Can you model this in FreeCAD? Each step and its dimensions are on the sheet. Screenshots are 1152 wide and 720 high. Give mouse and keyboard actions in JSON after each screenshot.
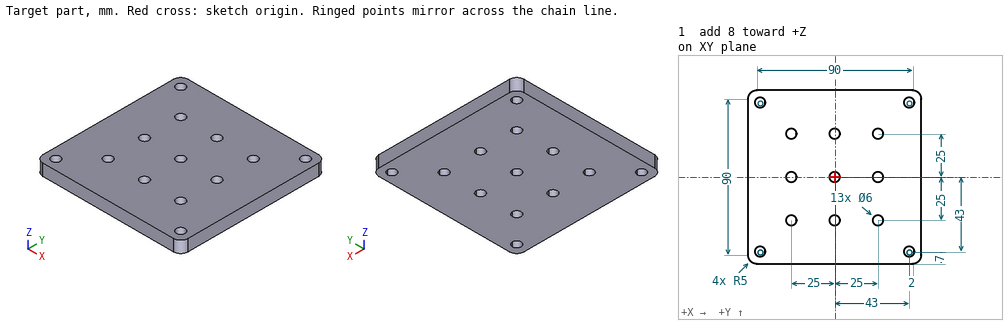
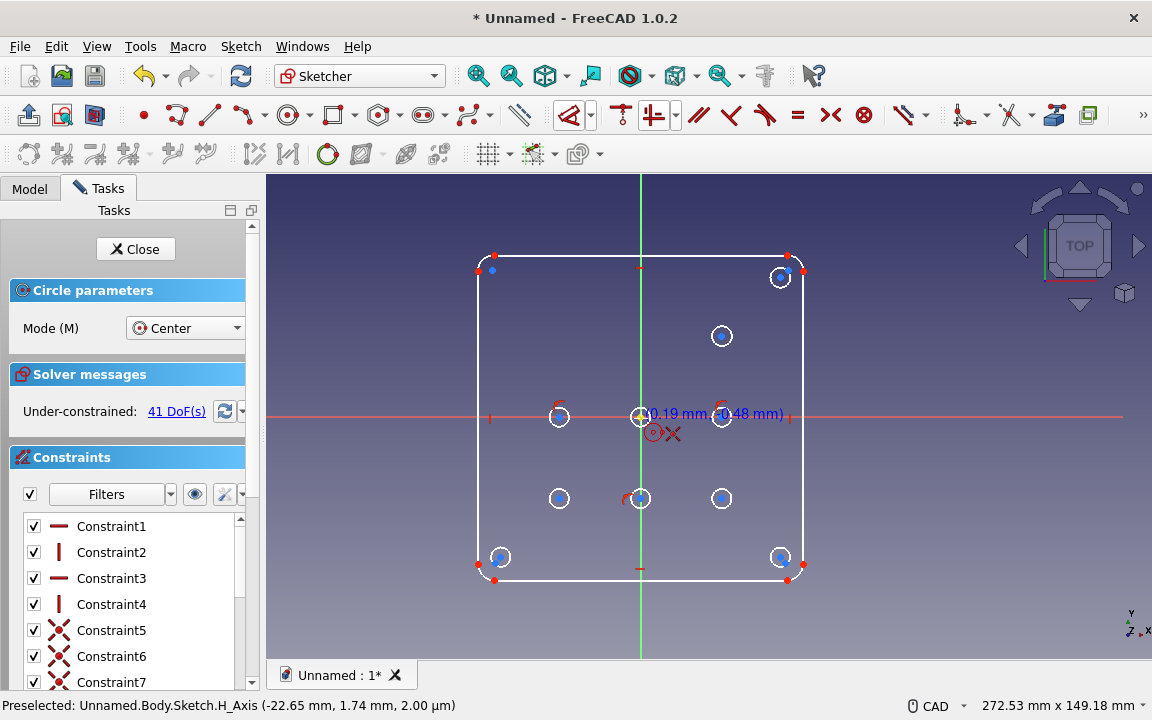
{"action": "scroll", "coordinate": [641, 336], "scroll_direction": "up", "scroll_amount": 5}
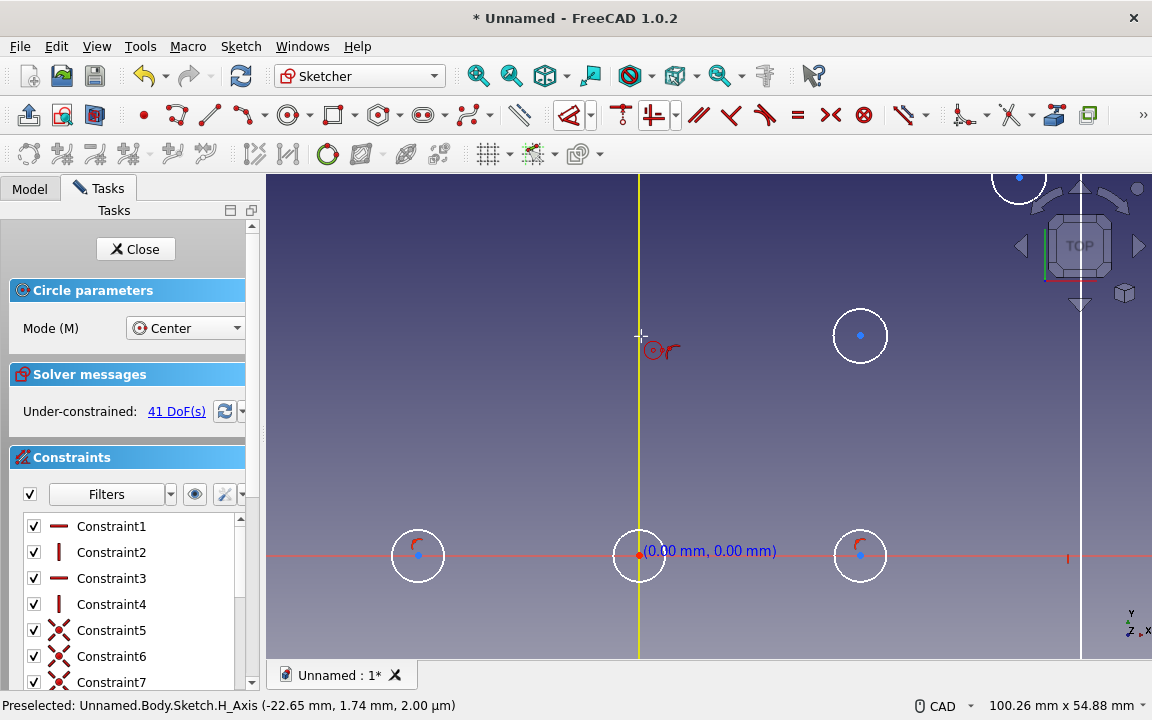
{"action": "left_click", "coordinate": [639, 335]}
{"action": "left_click", "coordinate": [658, 316]}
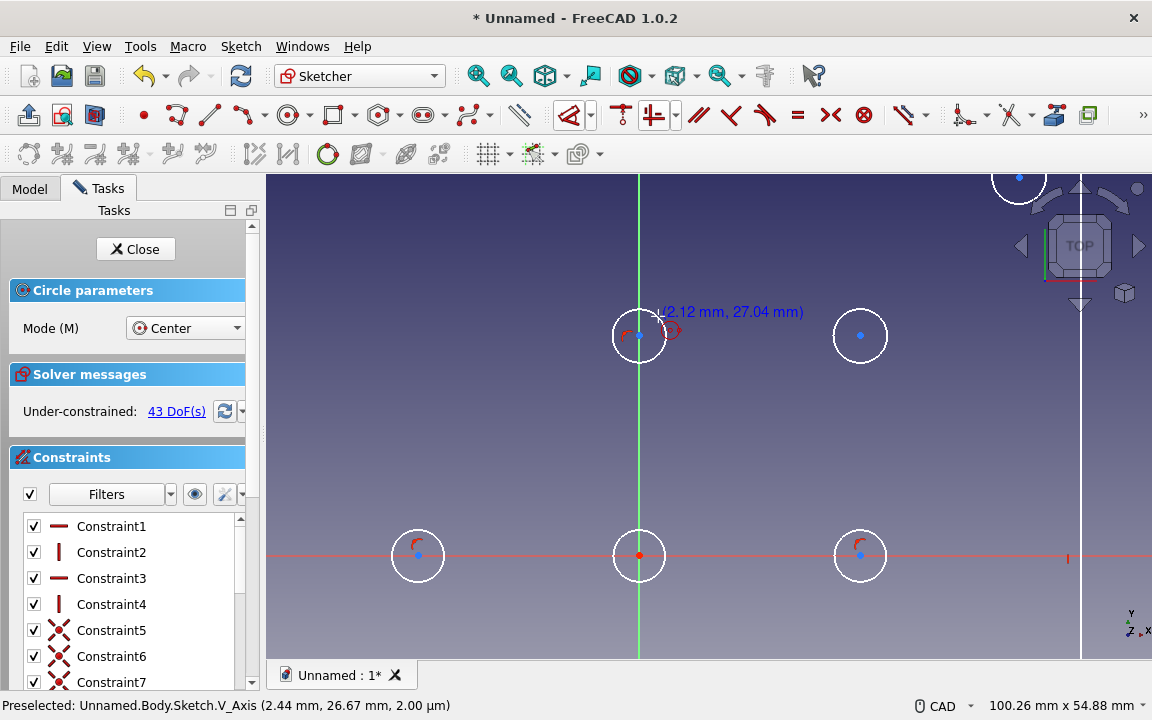
{"action": "left_click", "coordinate": [418, 335]}
{"action": "left_click", "coordinate": [437, 316]}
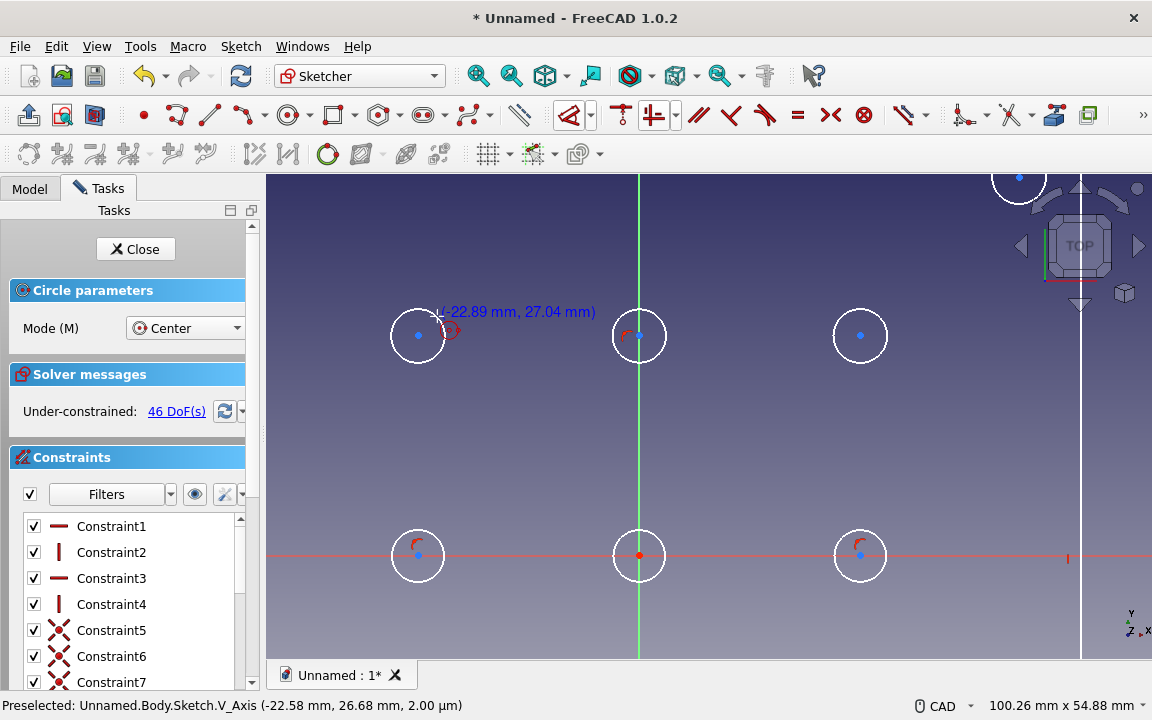
{"action": "scroll", "coordinate": [641, 335], "scroll_direction": "down", "scroll_amount": 5}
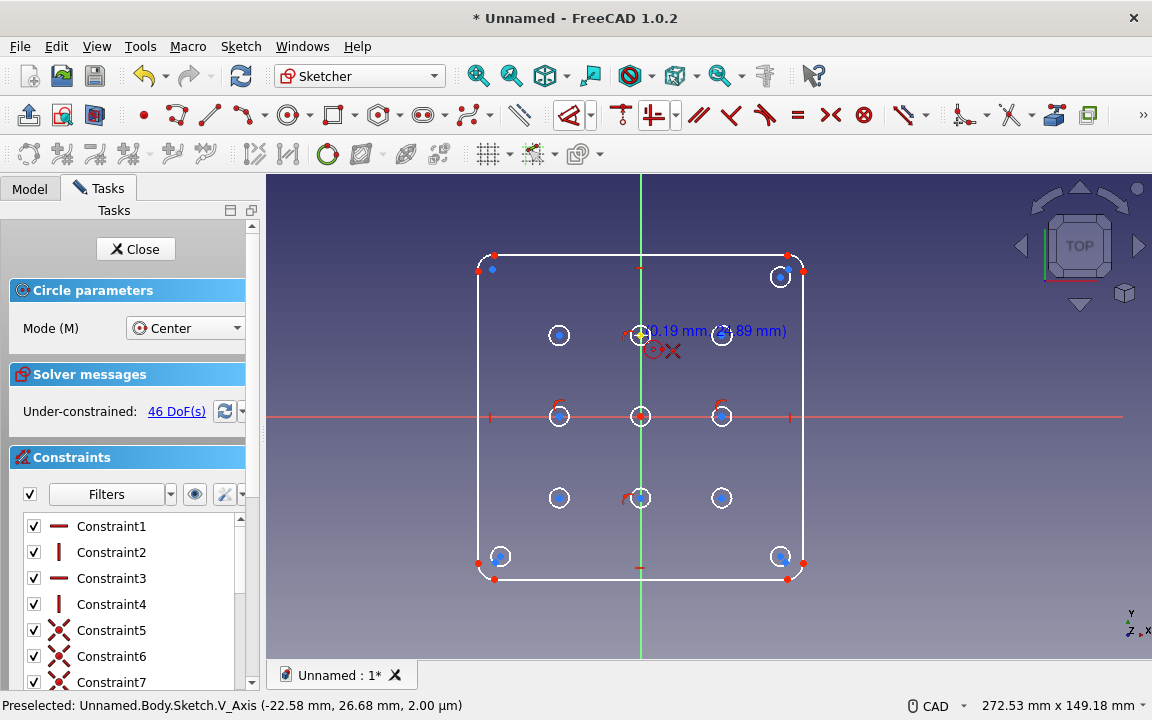
{"action": "scroll", "coordinate": [501, 277], "scroll_direction": "up", "scroll_amount": 5}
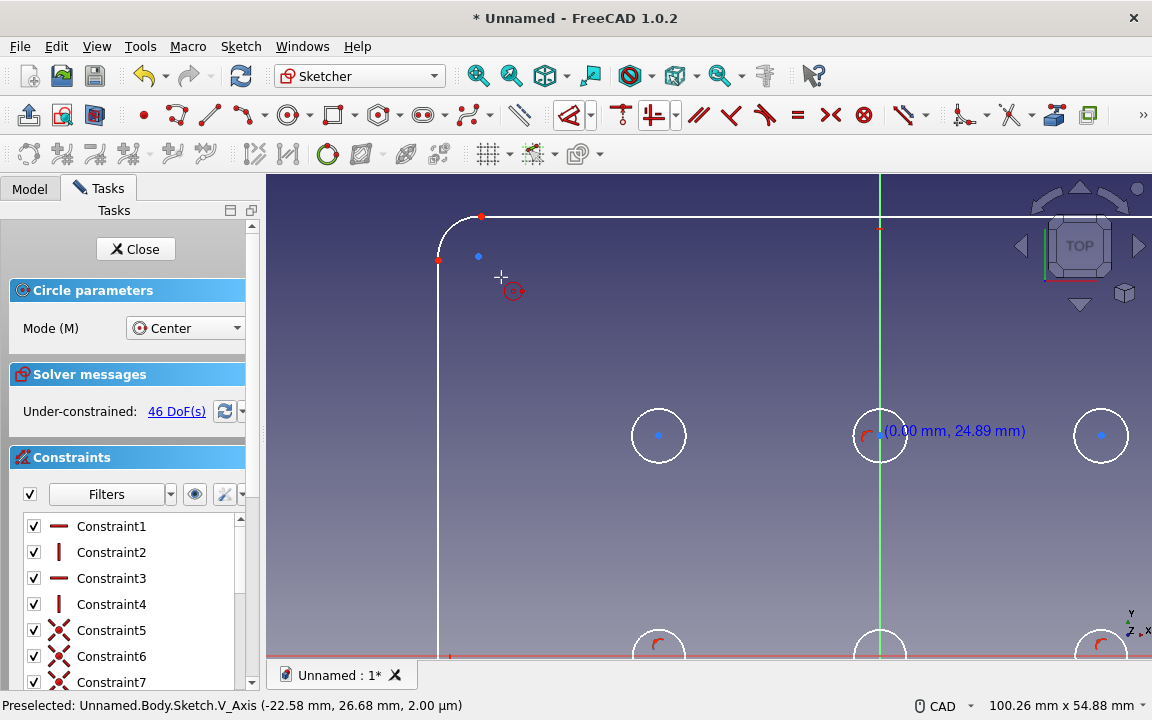
{"action": "left_click", "coordinate": [500, 276]}
{"action": "left_click", "coordinate": [519, 257]}
{"action": "key", "text": "Escape"}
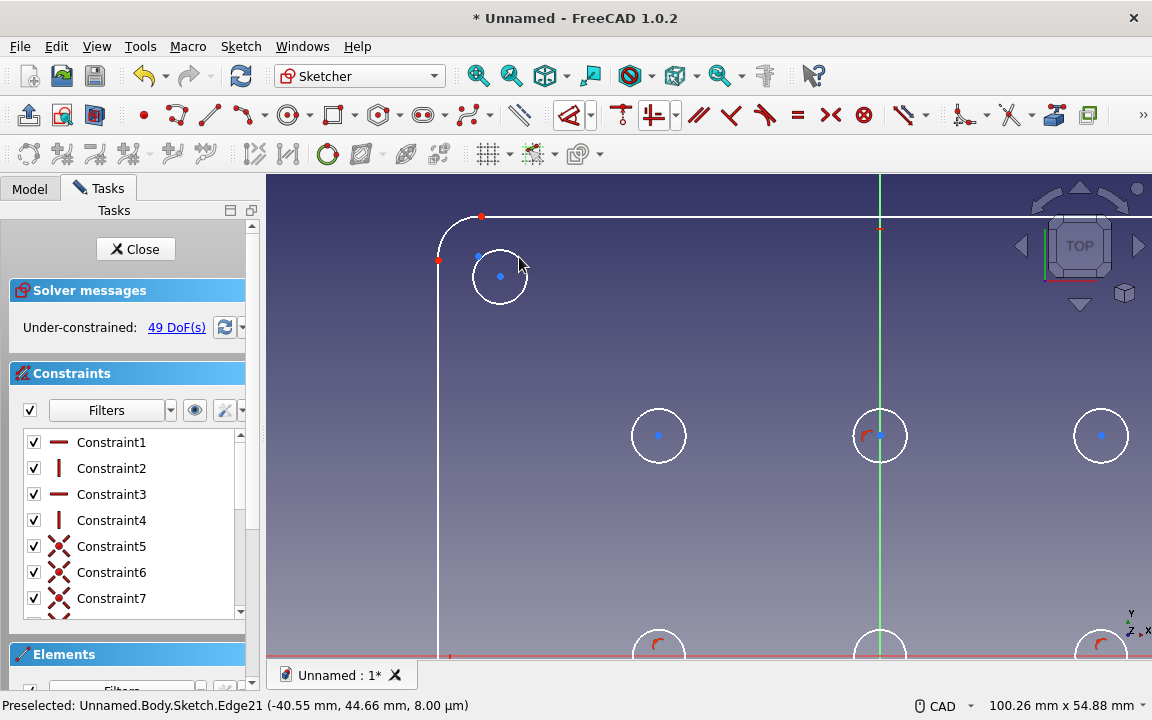
{"action": "left_click", "coordinate": [721, 217]}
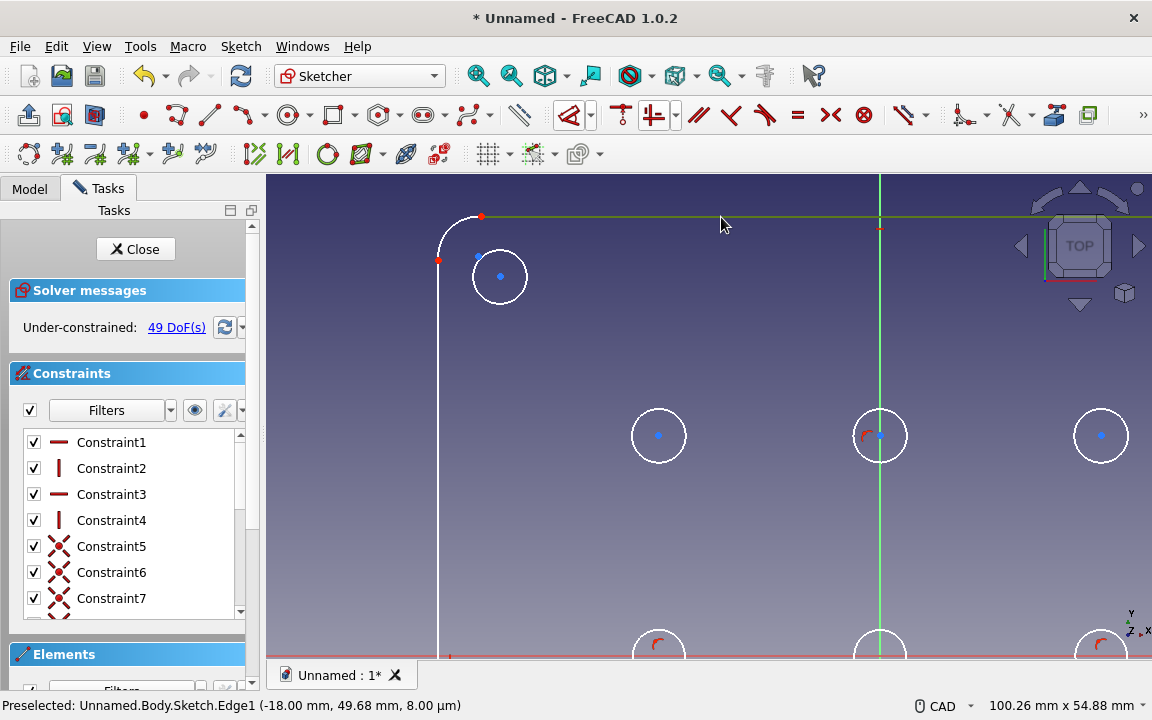
{"action": "left_click", "coordinate": [461, 220]}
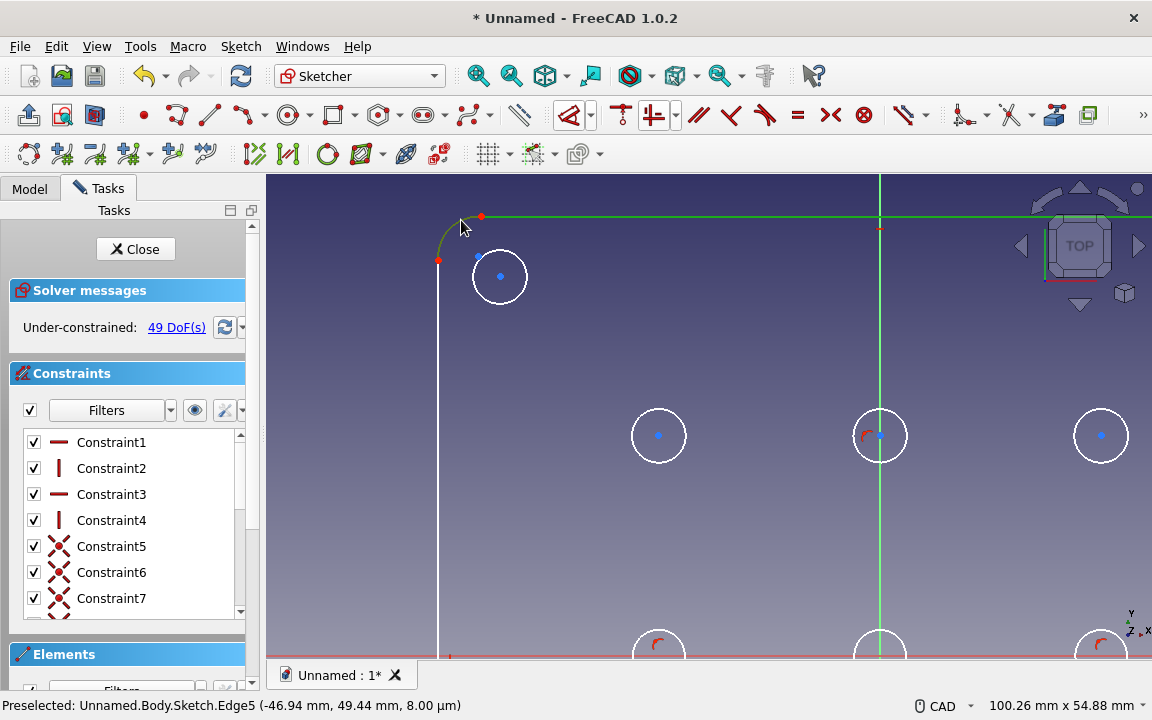
{"action": "left_click", "coordinate": [765, 116]}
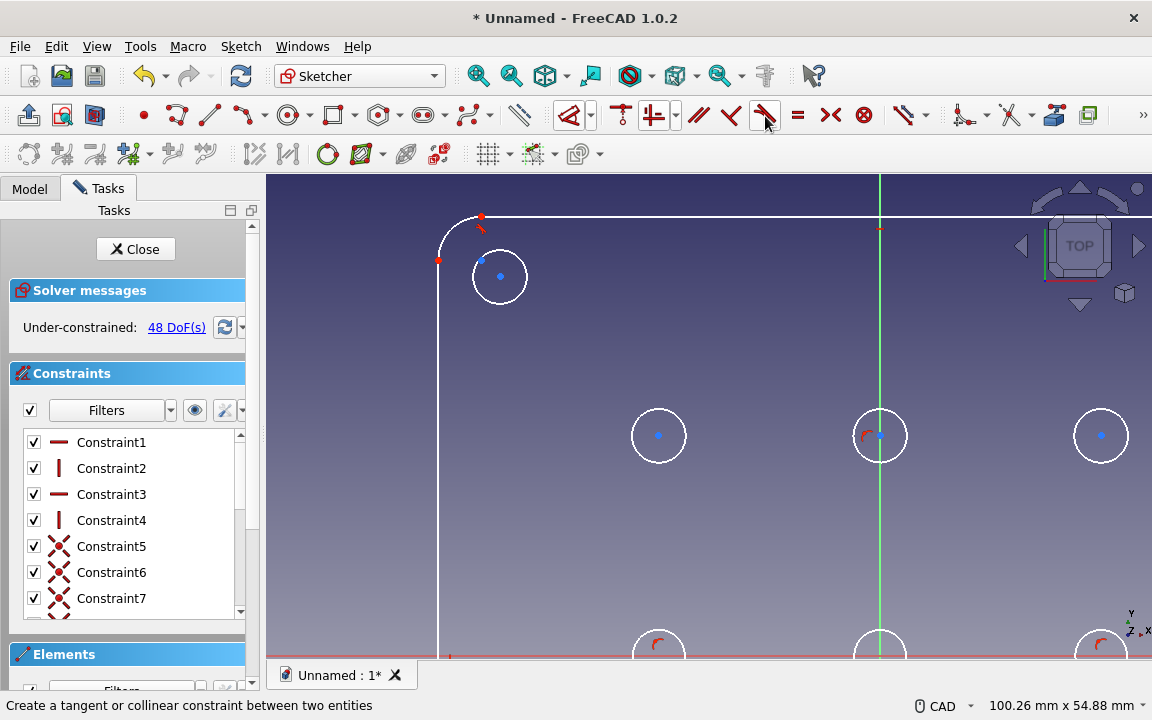
{"action": "left_click", "coordinate": [721, 217]}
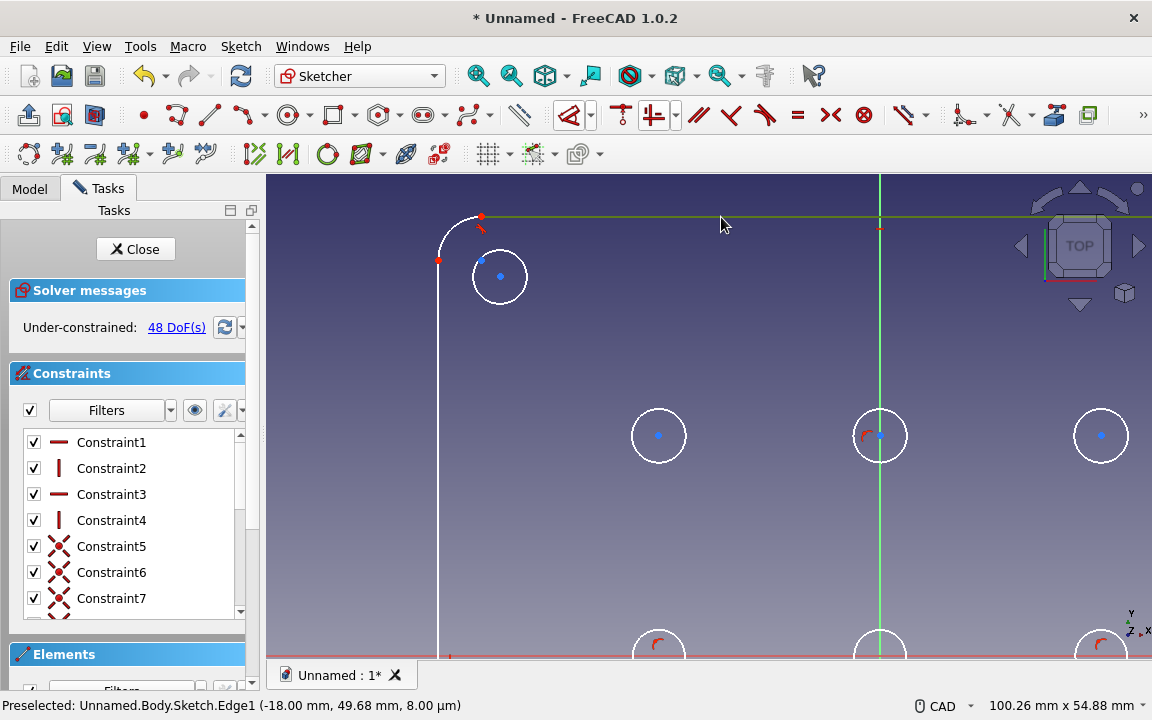
{"action": "scroll", "coordinate": [501, 277], "scroll_direction": "down", "scroll_amount": 5}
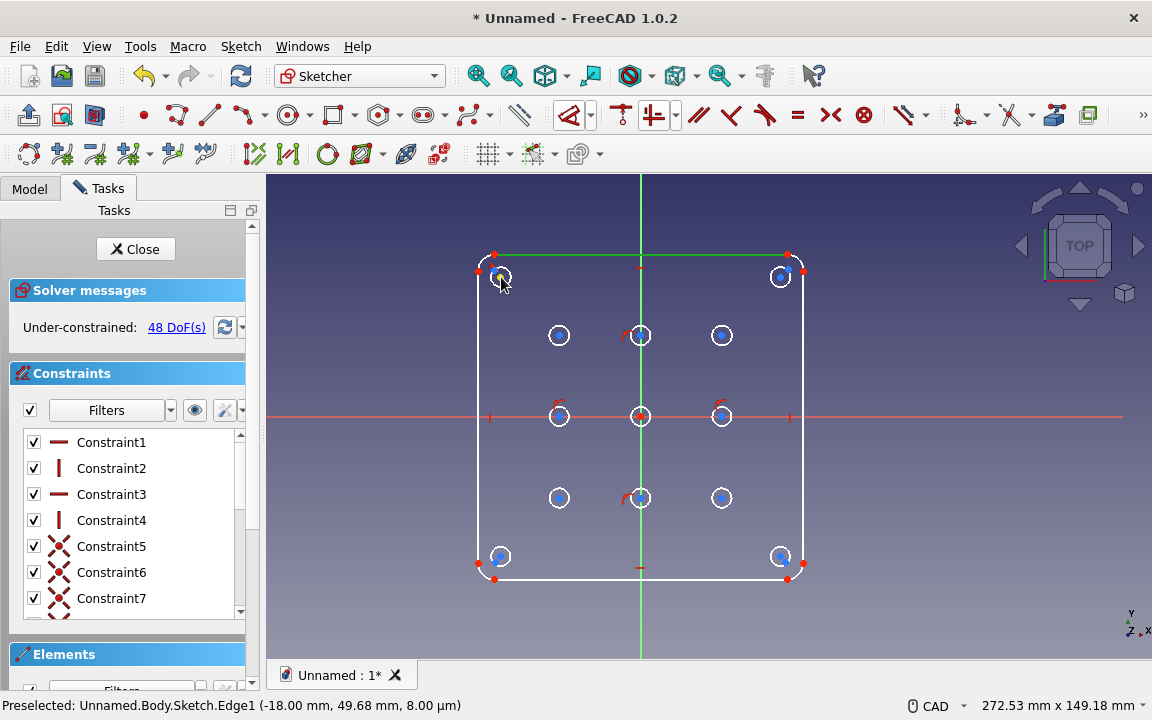
{"action": "scroll", "coordinate": [802, 264], "scroll_direction": "up", "scroll_amount": 3}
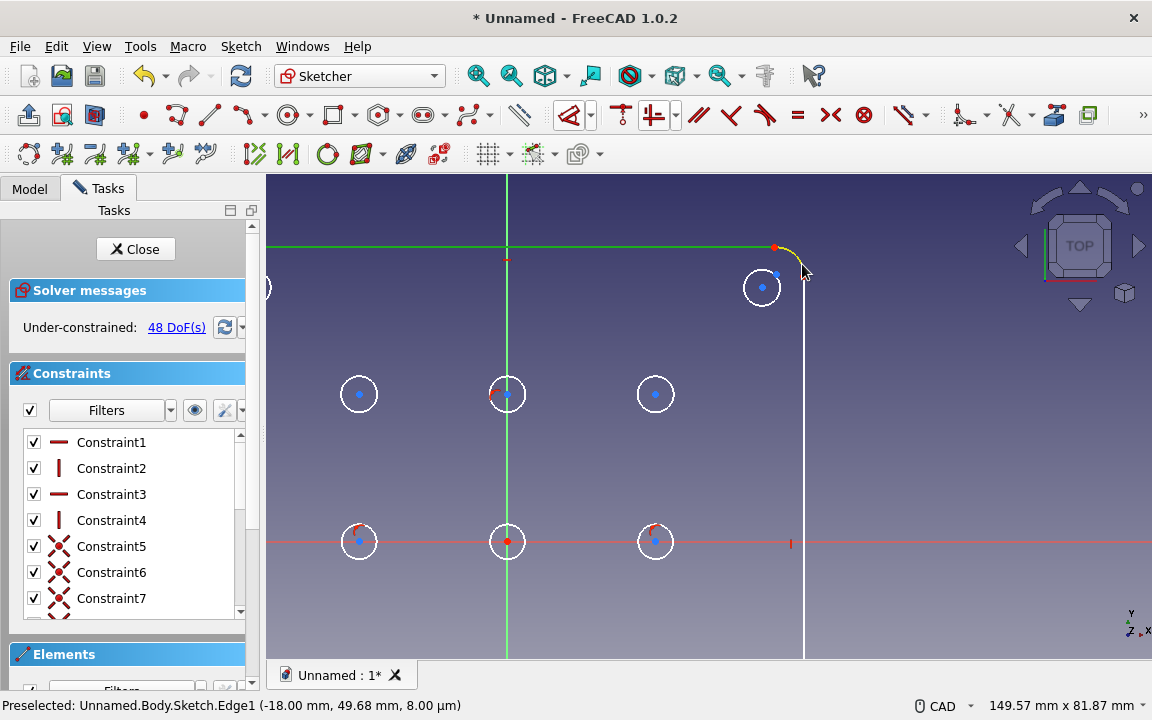
{"action": "left_click", "coordinate": [801, 263]}